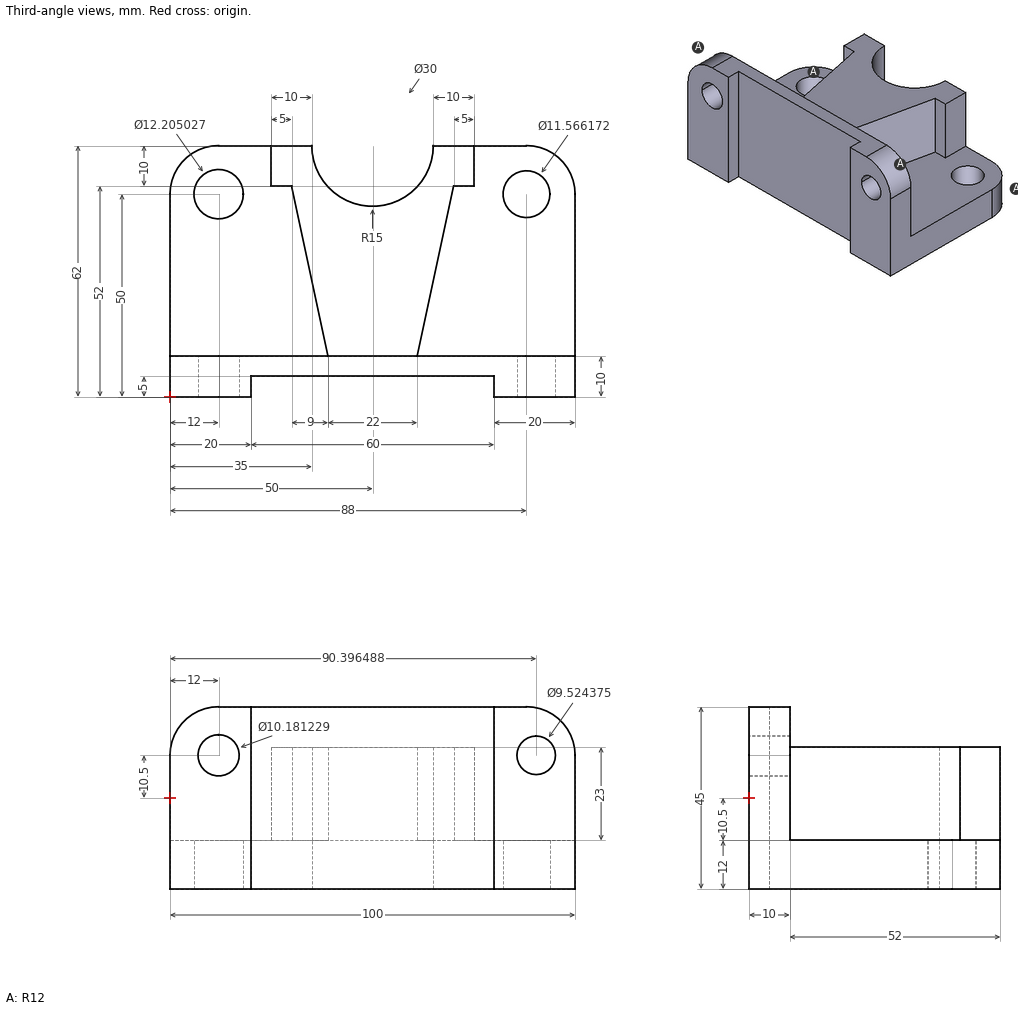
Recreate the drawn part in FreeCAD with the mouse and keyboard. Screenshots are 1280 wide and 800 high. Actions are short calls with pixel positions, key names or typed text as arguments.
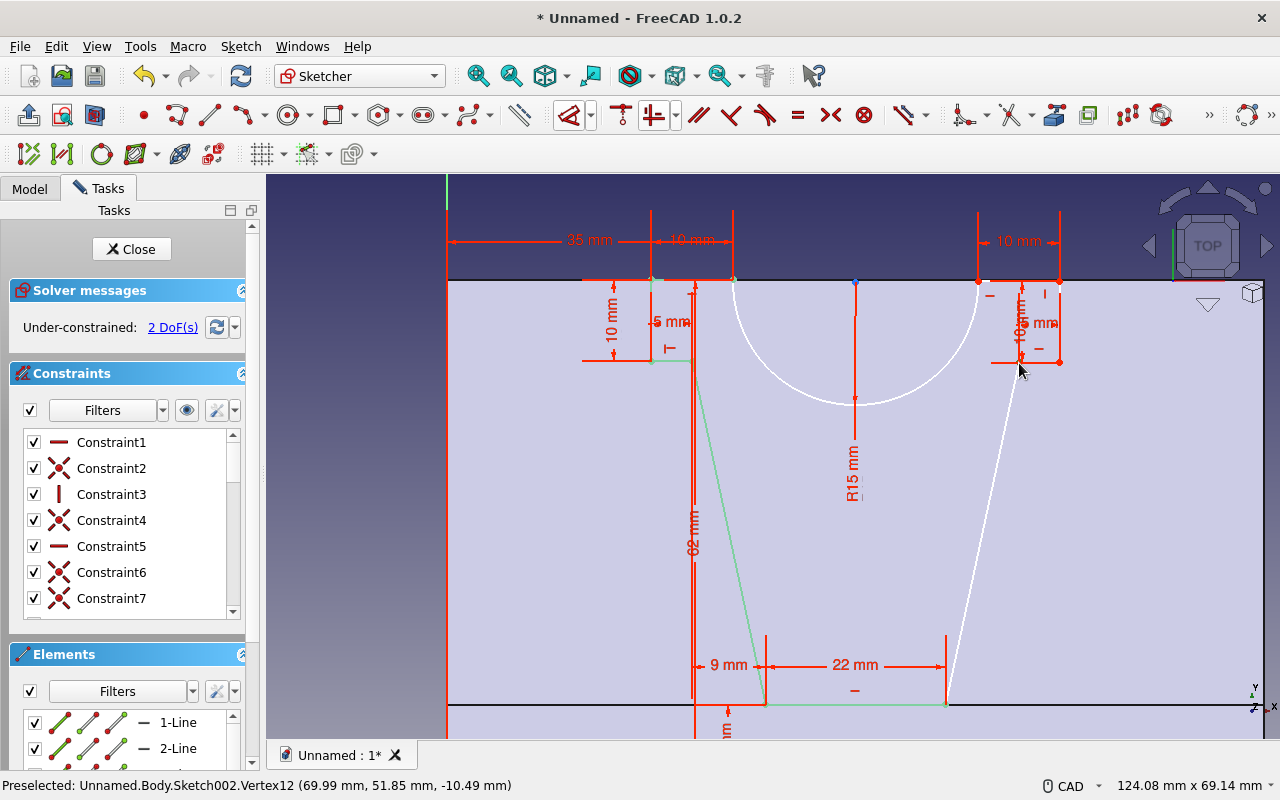
key(i)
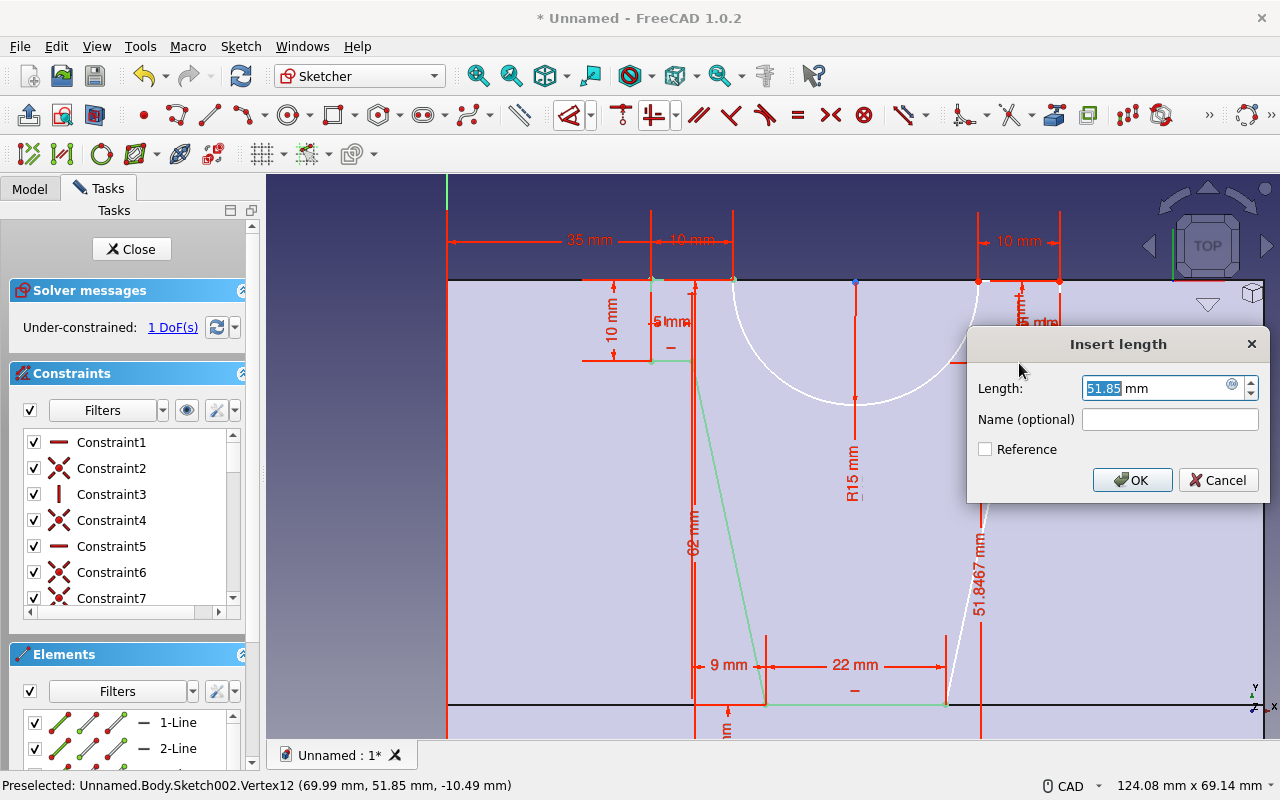
text(52)
key(Return)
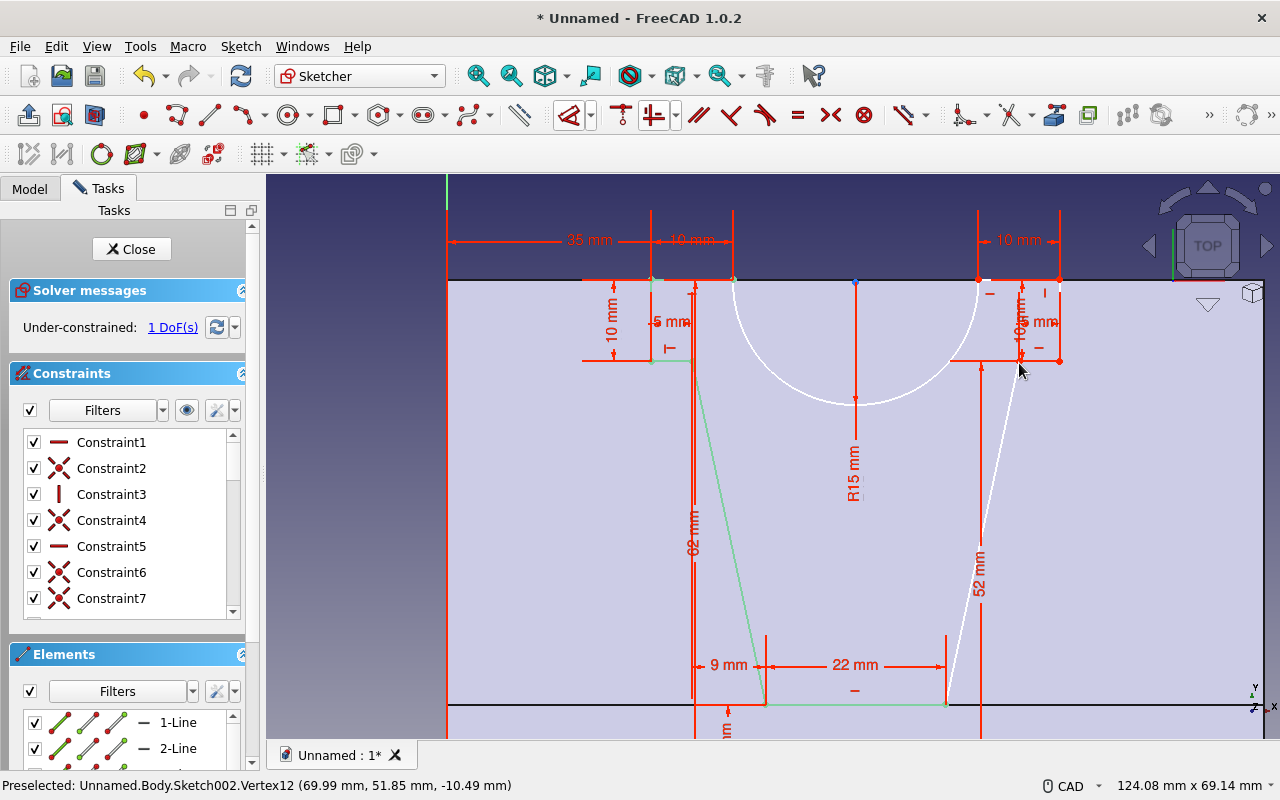
click(856, 283)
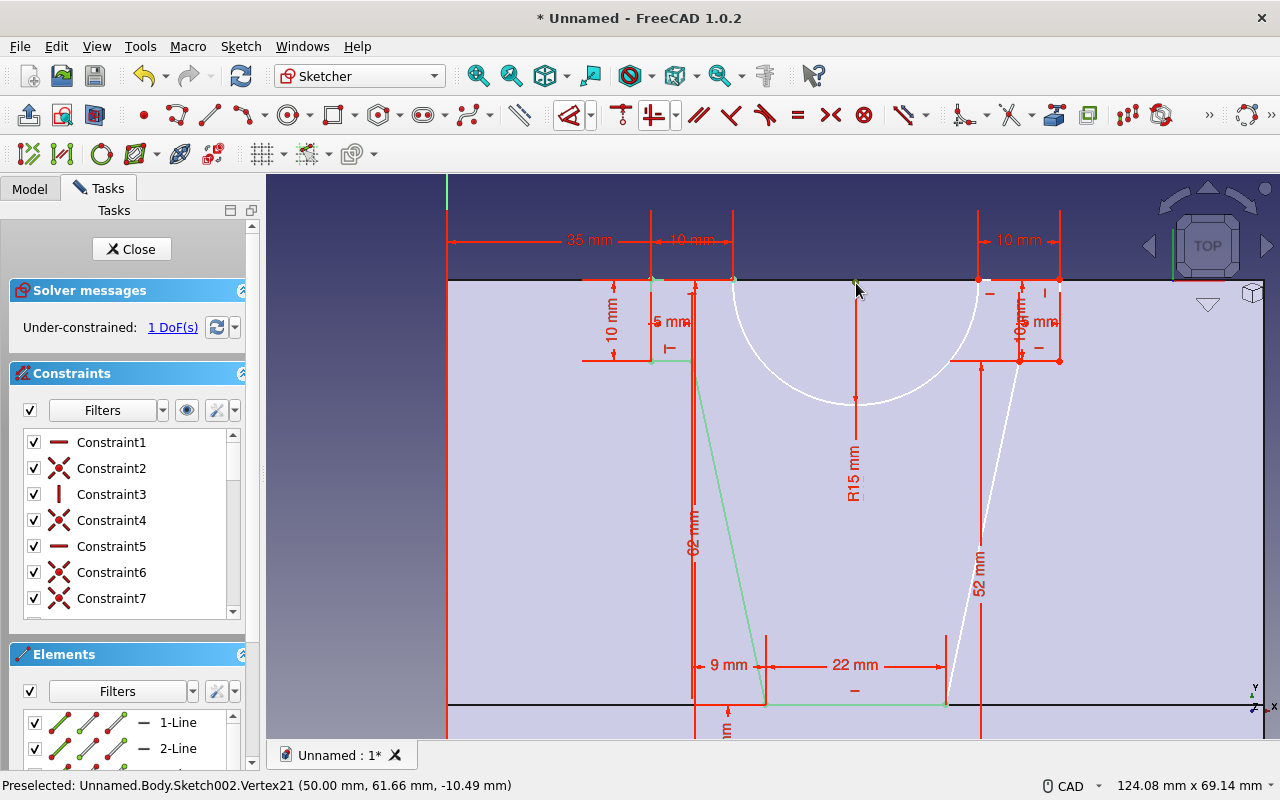
key(i)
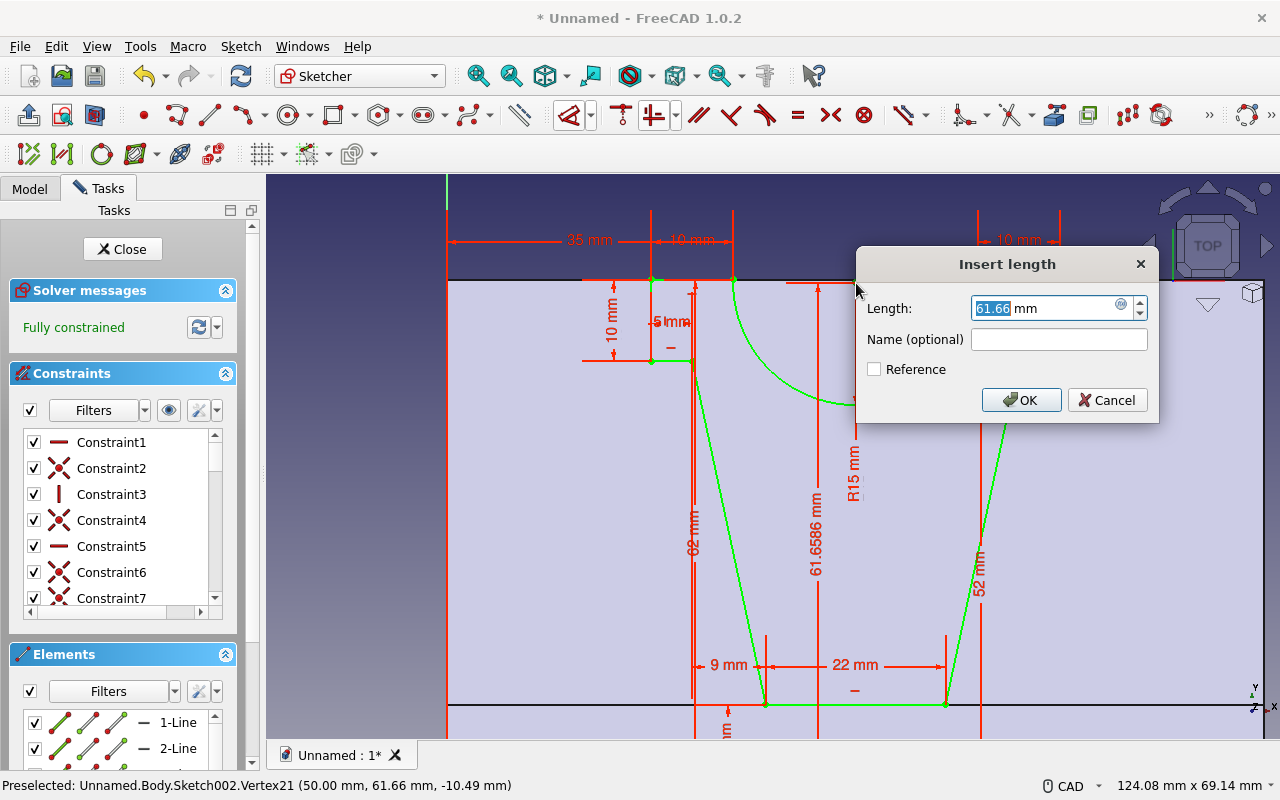
text(62)
key(Return)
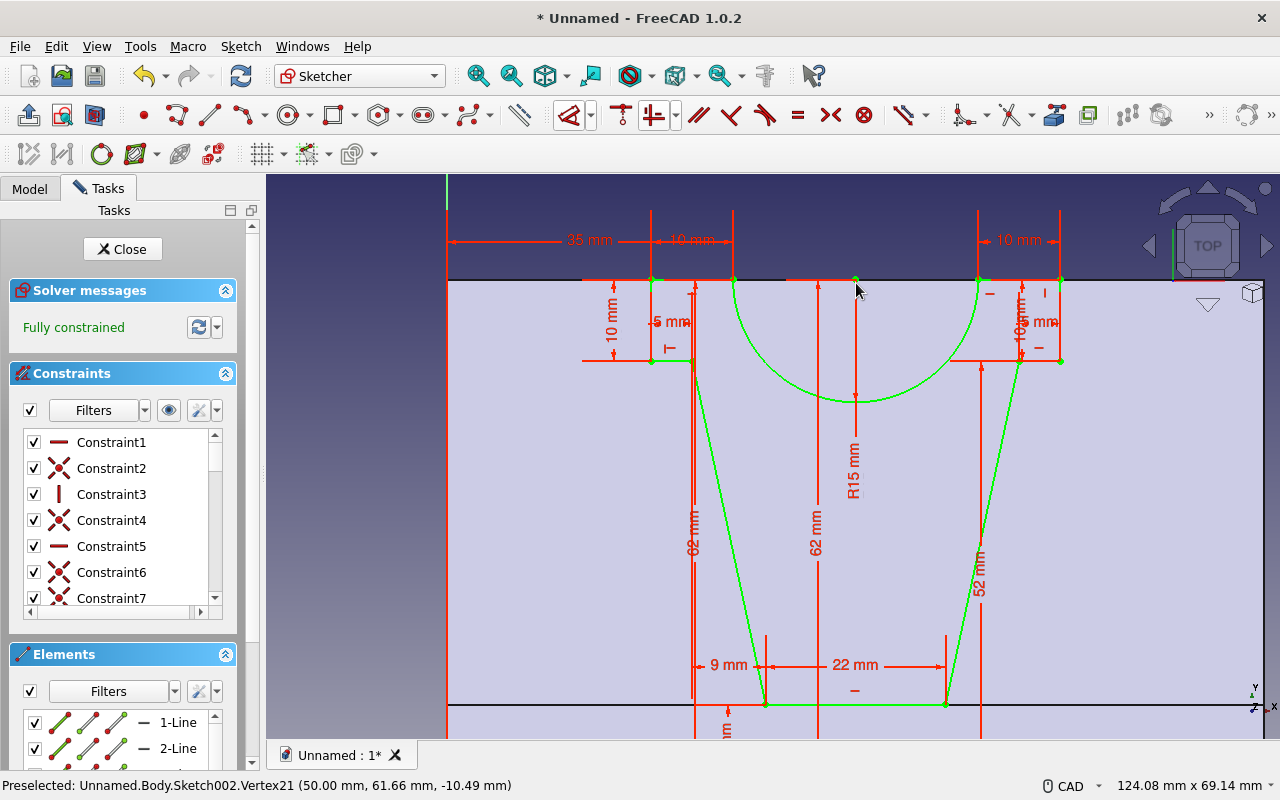
click(123, 249)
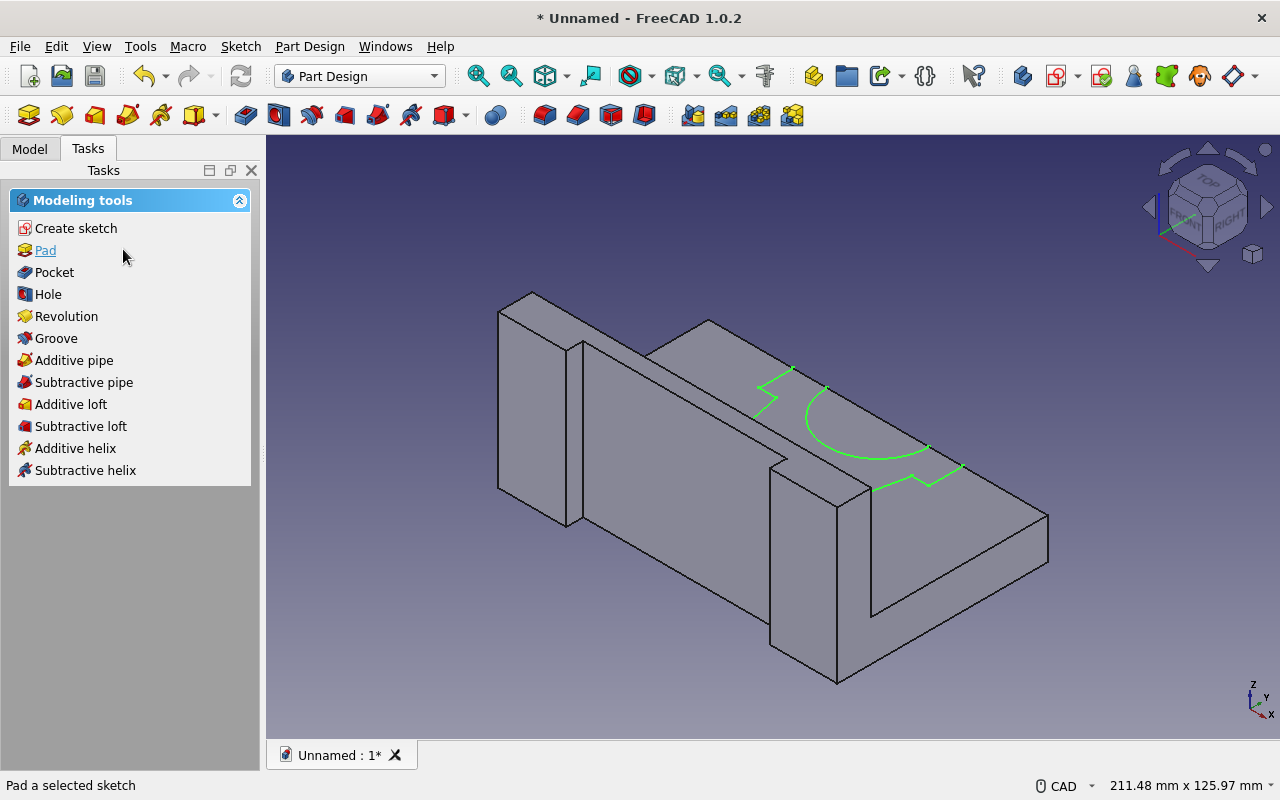
click(29, 116)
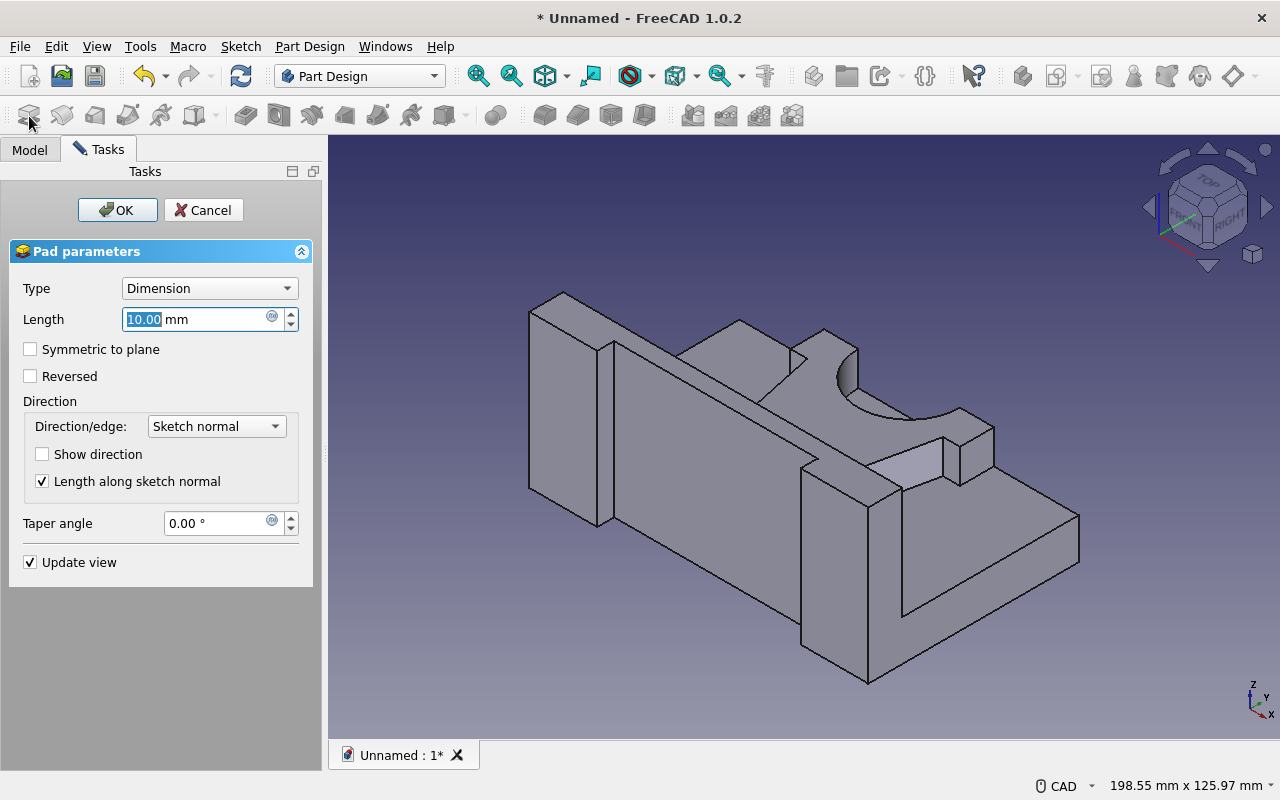
text(23)
key(Tab)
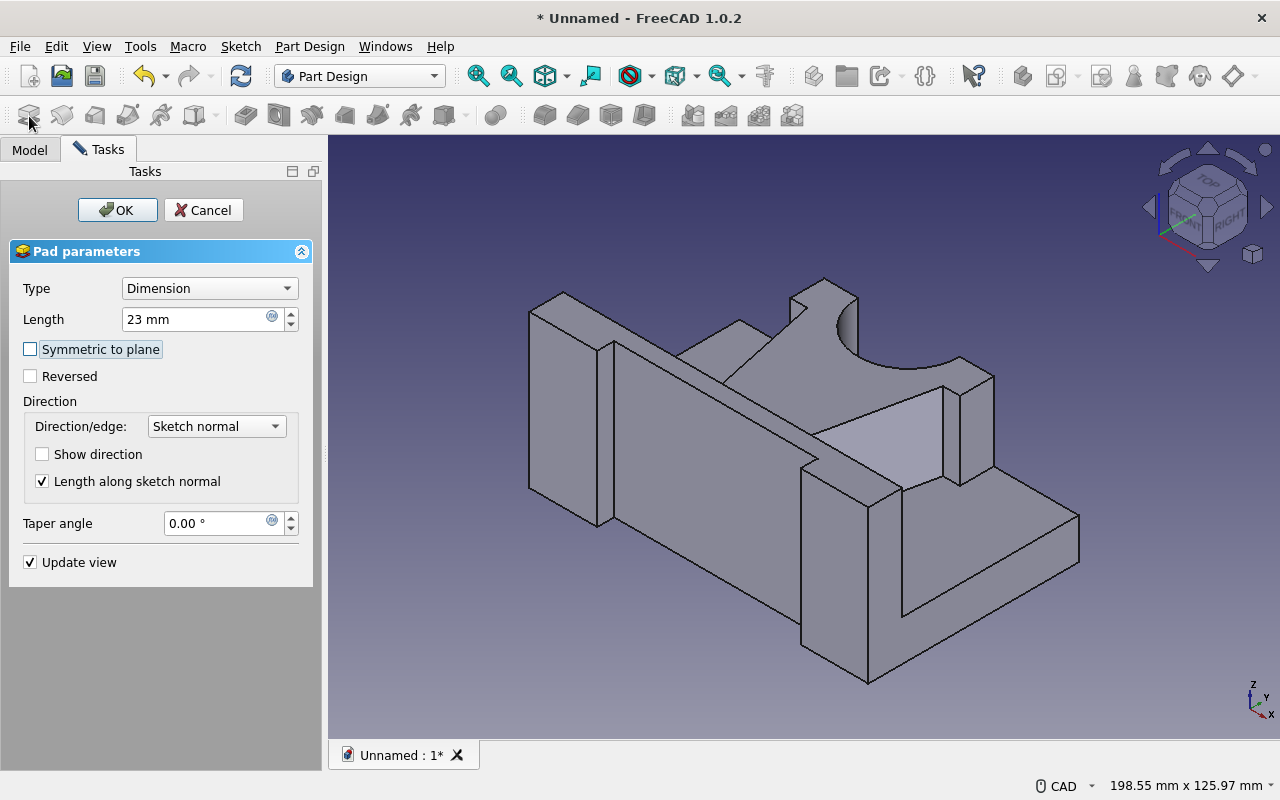
click(118, 210)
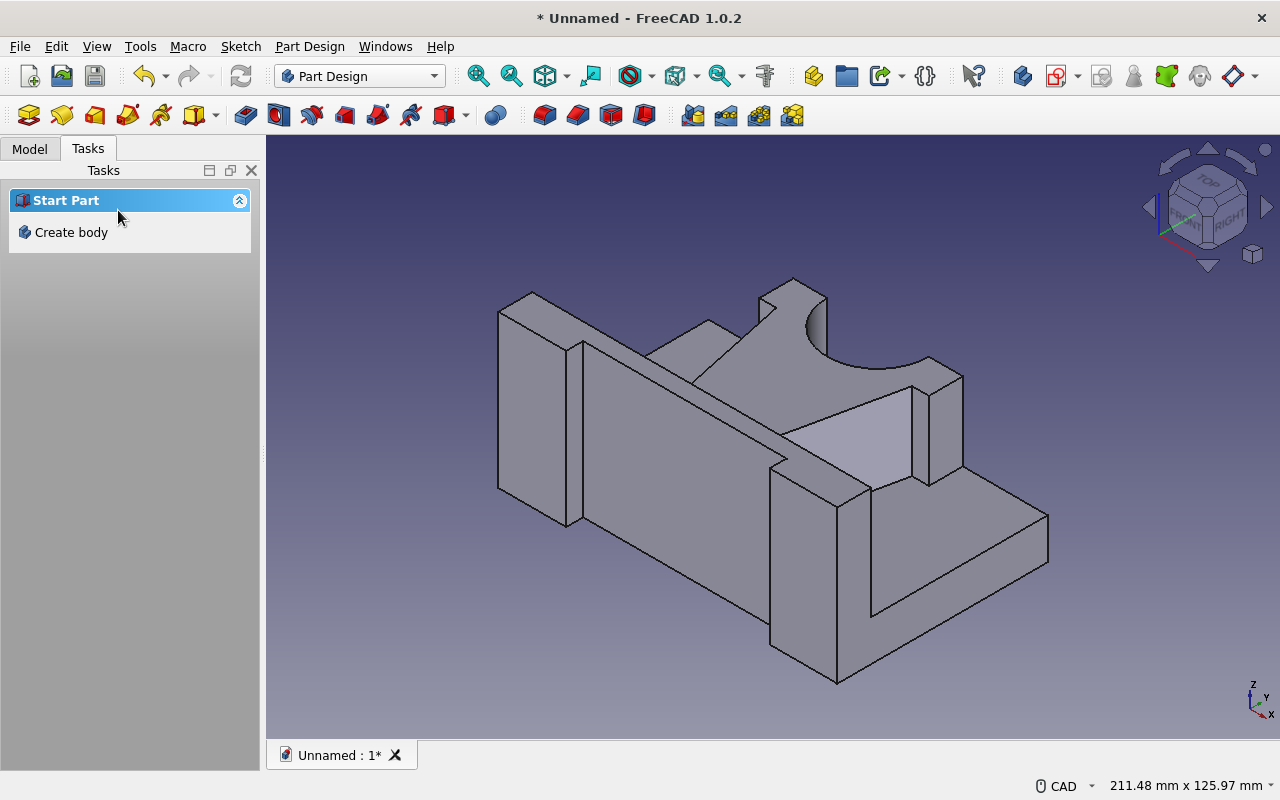
click(937, 523)